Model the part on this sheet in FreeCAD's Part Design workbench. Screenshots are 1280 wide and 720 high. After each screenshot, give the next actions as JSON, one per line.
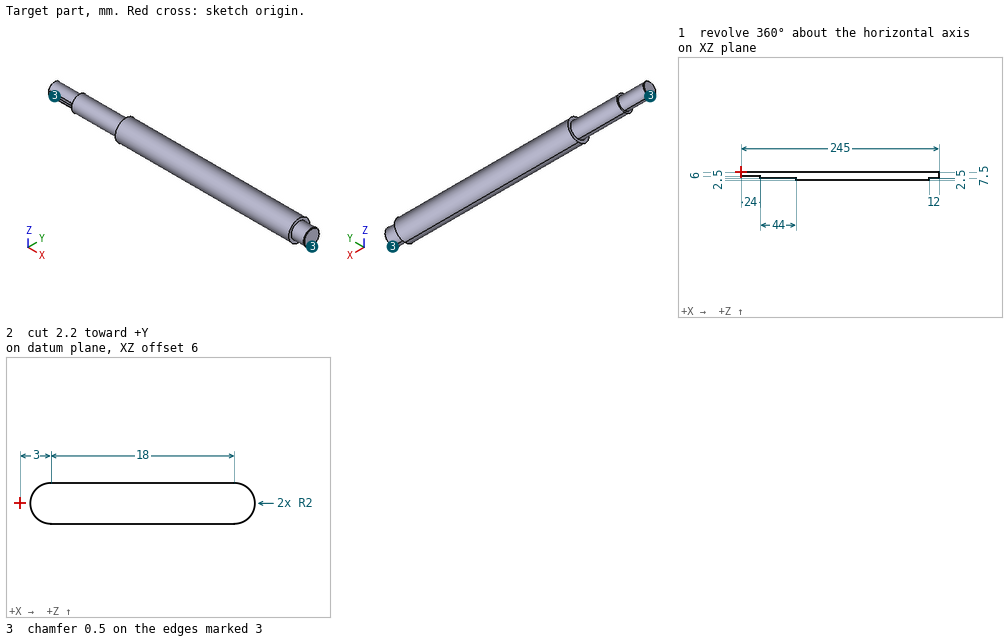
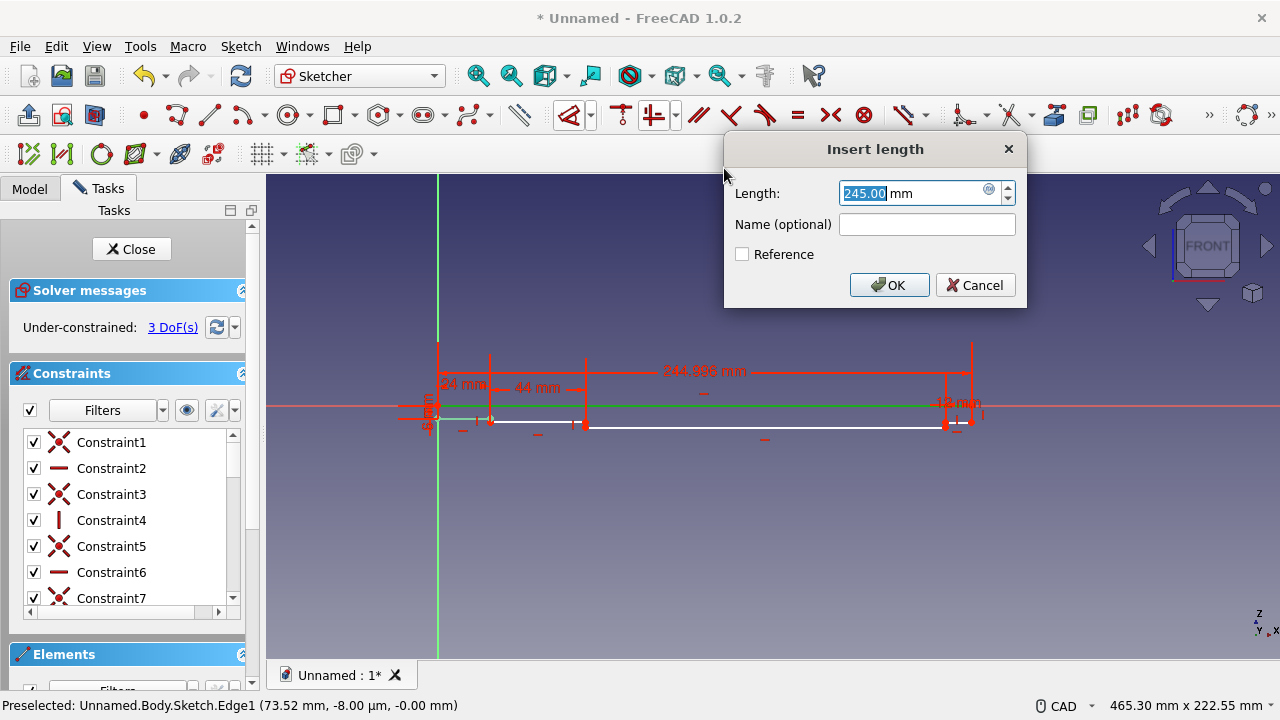
{"action": "type", "text": "245"}
{"action": "key", "text": "Return"}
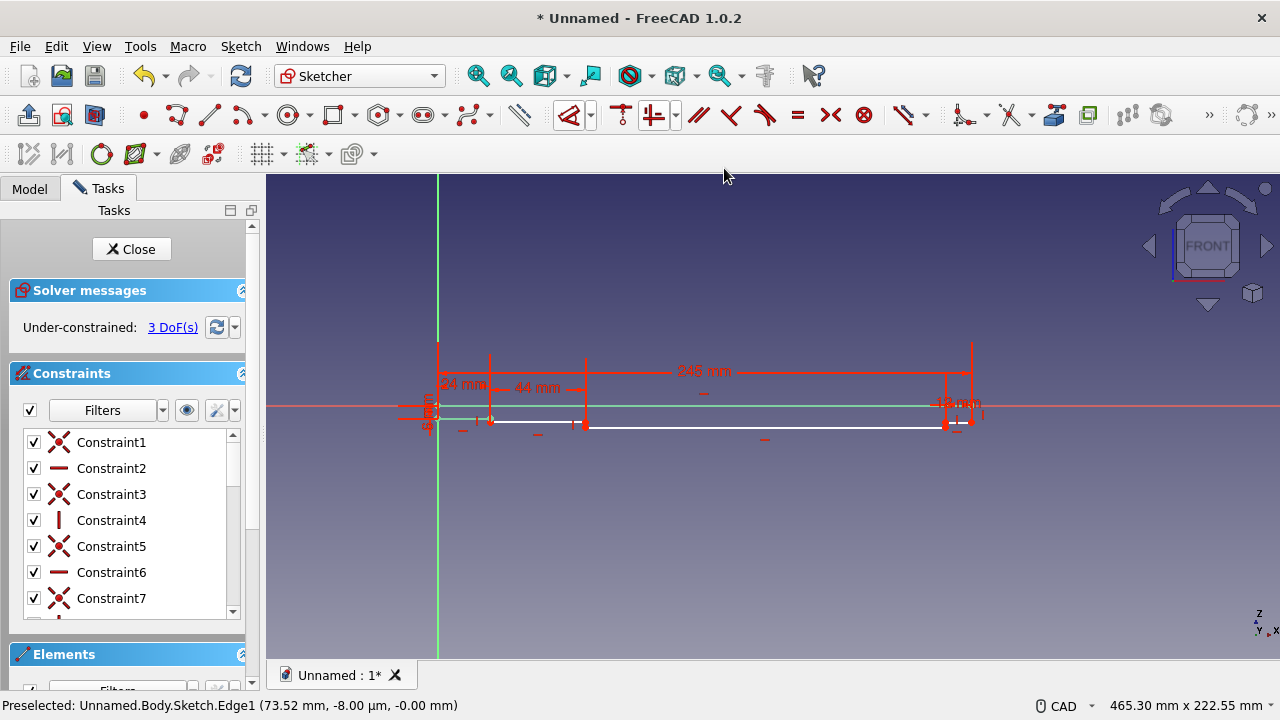
{"action": "scroll", "coordinate": [972, 414], "scroll_direction": "up", "scroll_amount": 5}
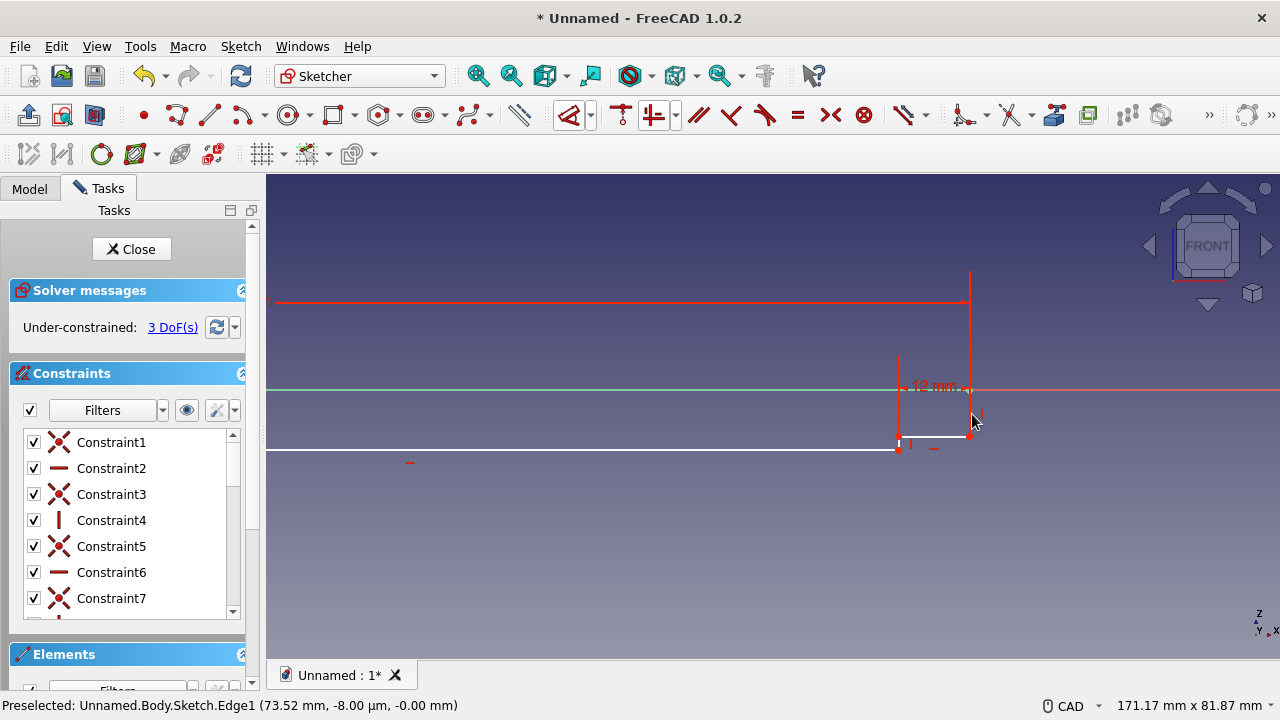
{"action": "left_click", "coordinate": [970, 414]}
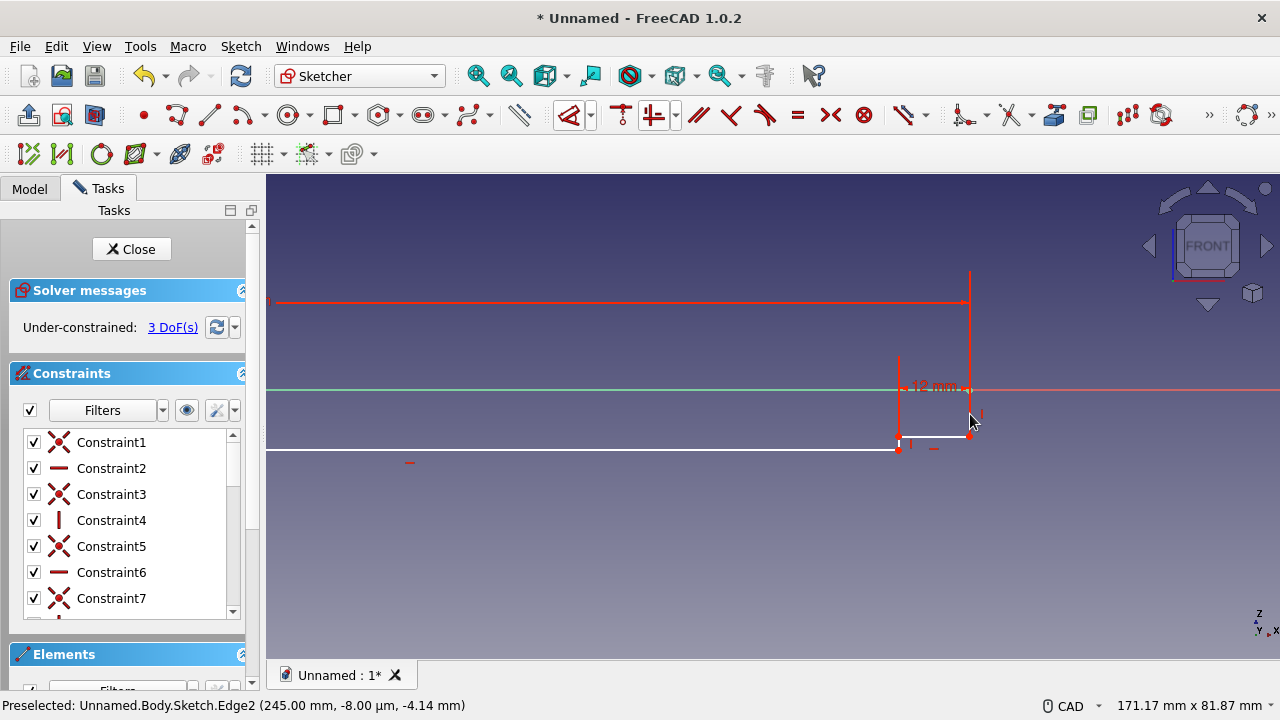
{"action": "left_click", "coordinate": [590, 116]}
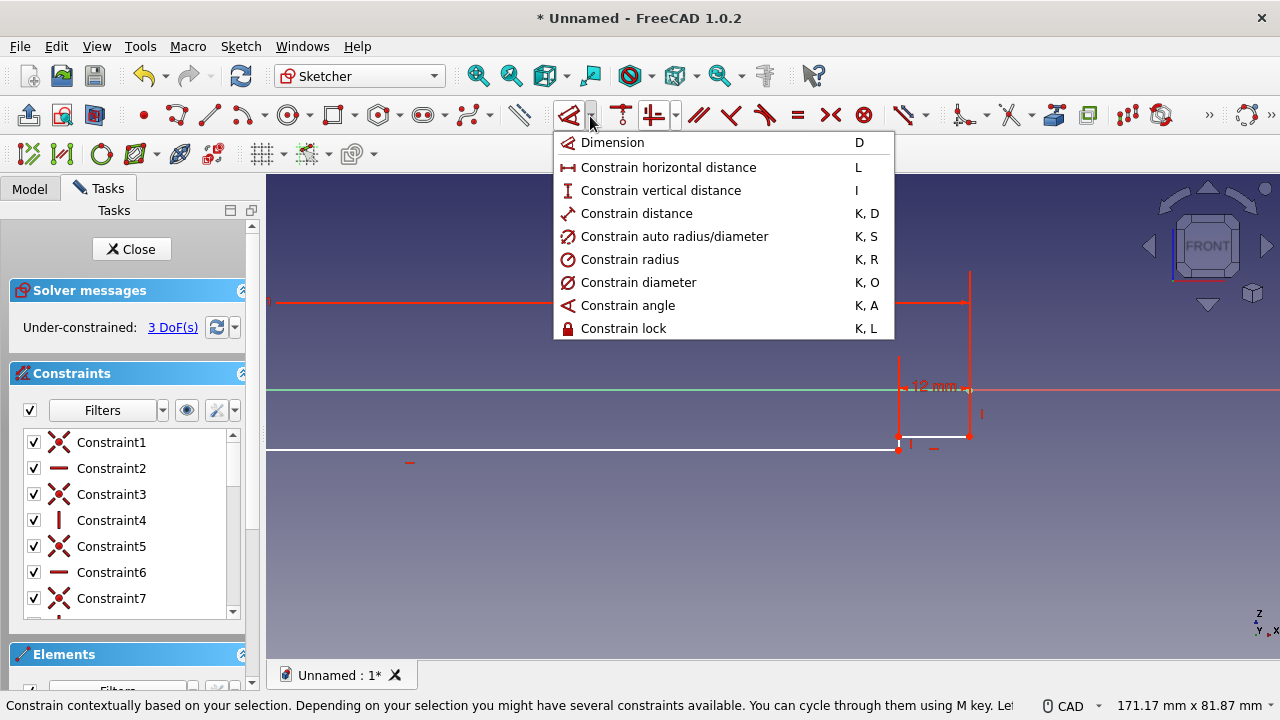
{"action": "left_click", "coordinate": [724, 190]}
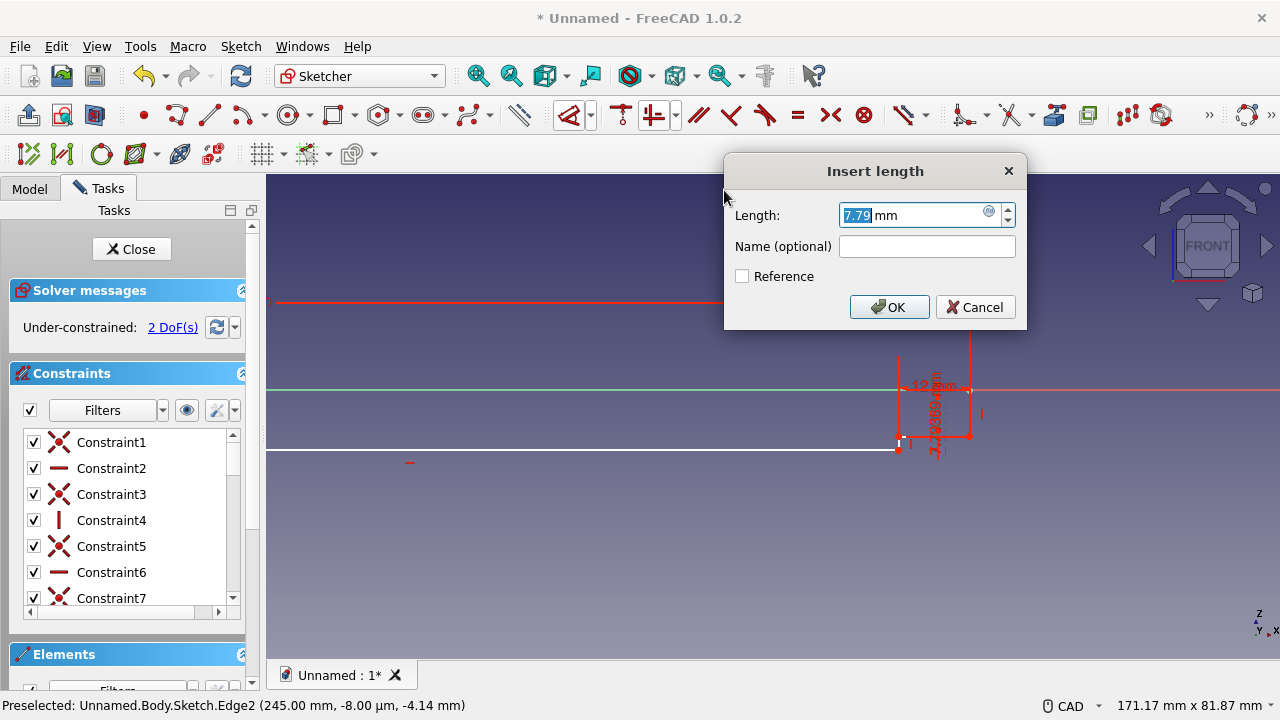
{"action": "type", "text": "7.5"}
{"action": "key", "text": "Return"}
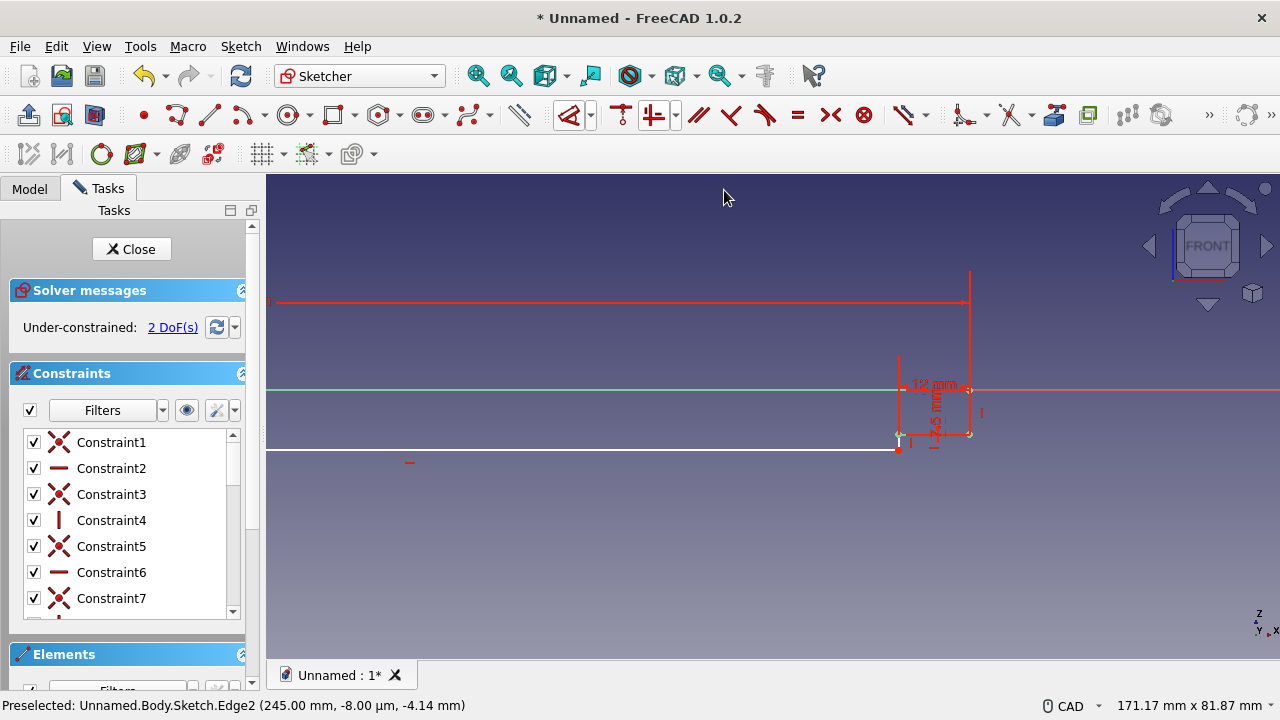
{"action": "scroll", "coordinate": [899, 443], "scroll_direction": "up", "scroll_amount": 5}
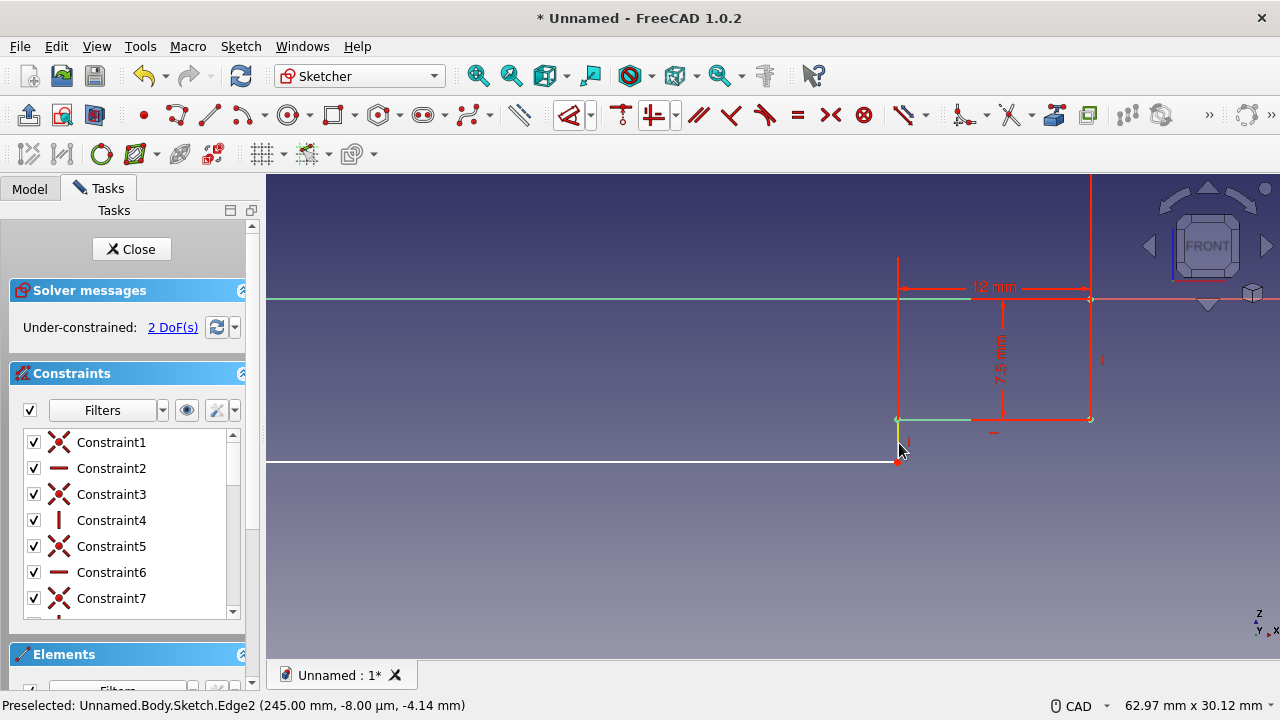
{"action": "left_click", "coordinate": [898, 441]}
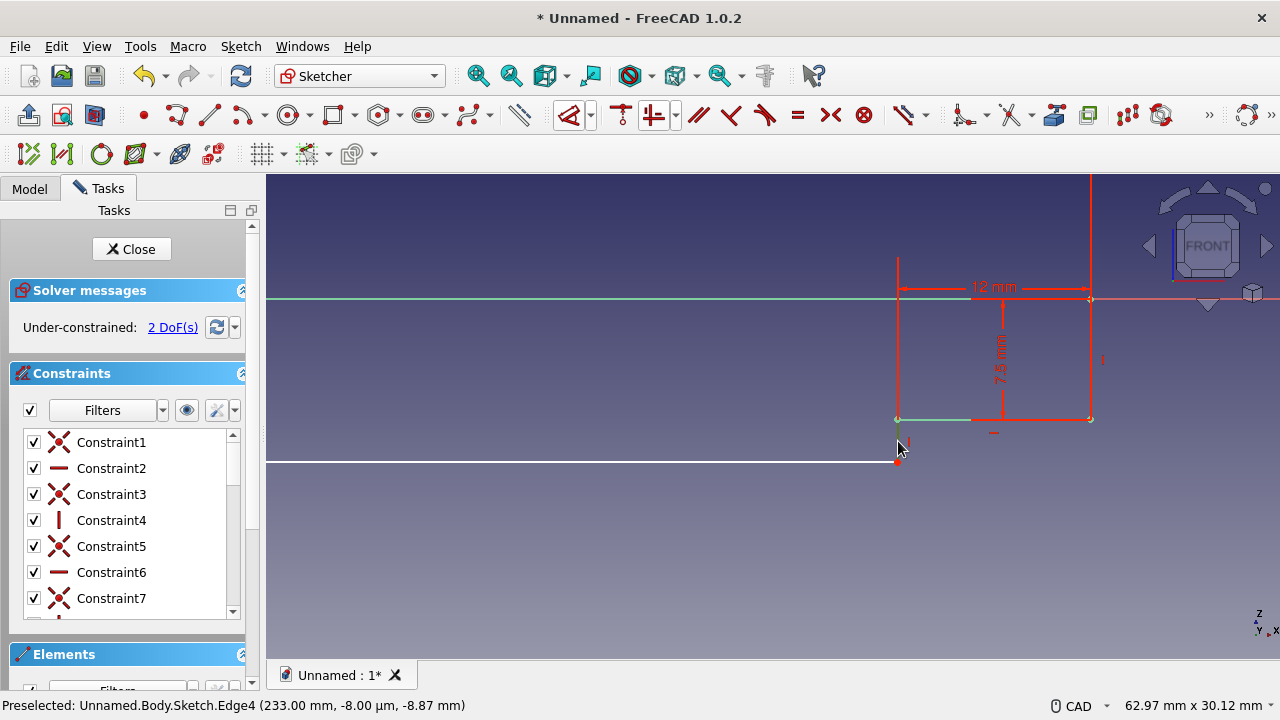
{"action": "left_click", "coordinate": [590, 116]}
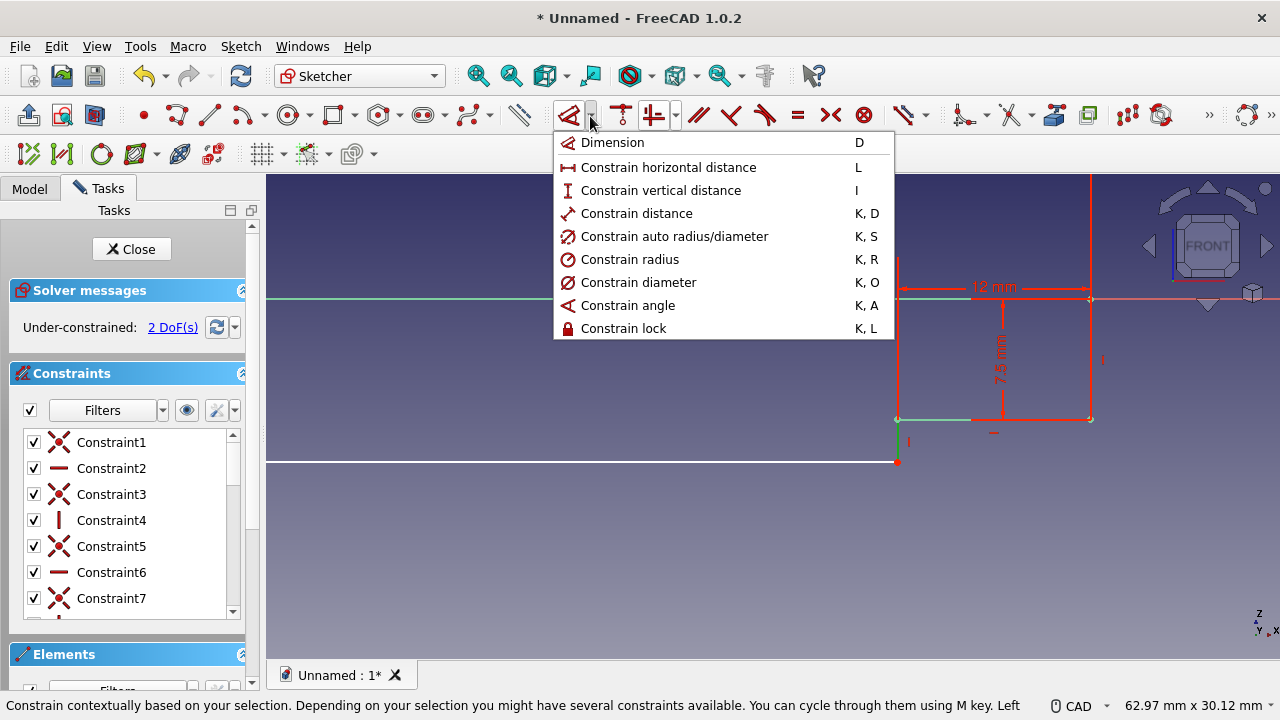
{"action": "left_click", "coordinate": [724, 190]}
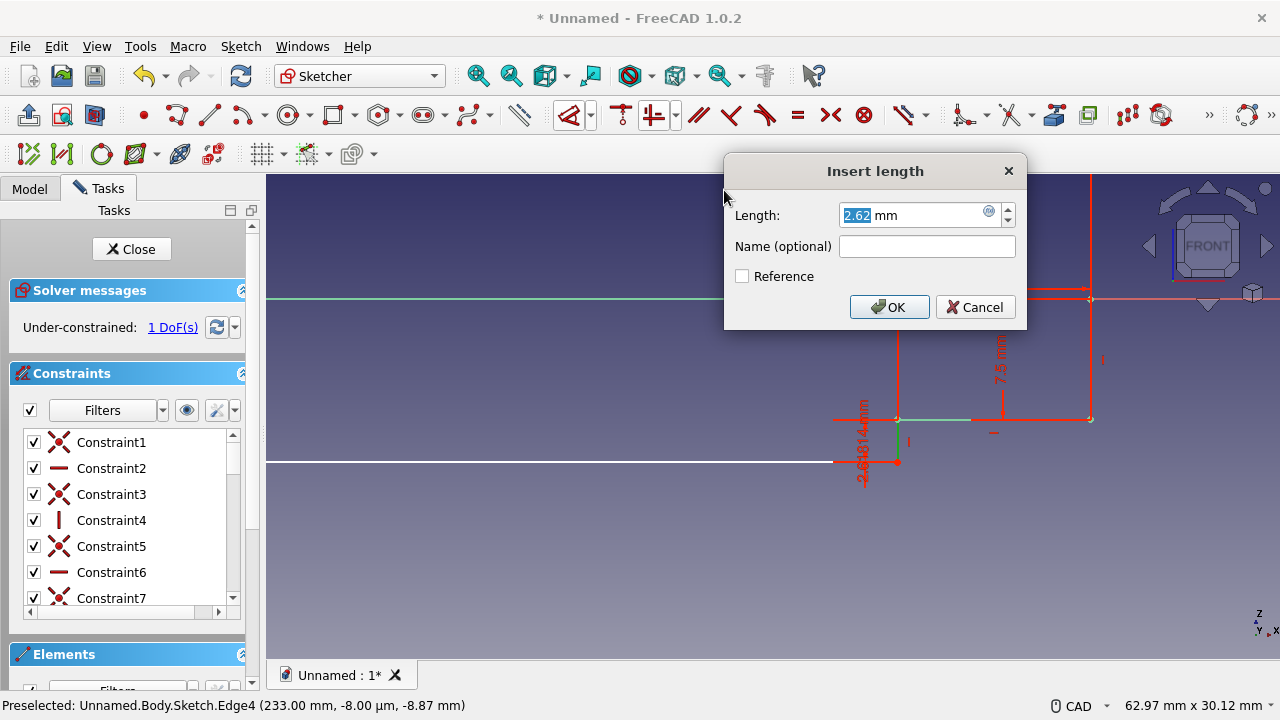
{"action": "type", "text": "2.5"}
{"action": "key", "text": "Return"}